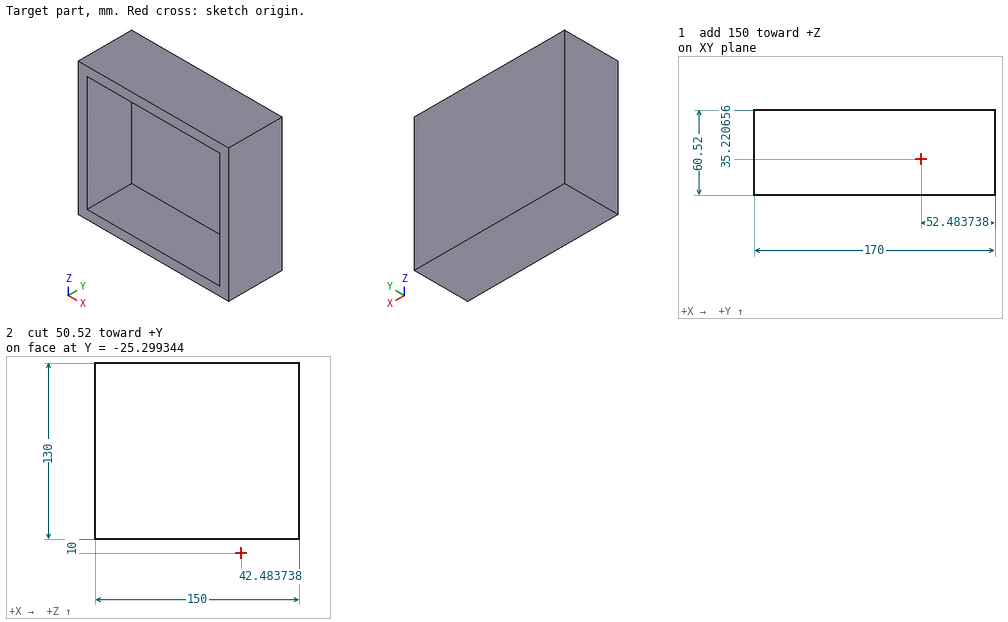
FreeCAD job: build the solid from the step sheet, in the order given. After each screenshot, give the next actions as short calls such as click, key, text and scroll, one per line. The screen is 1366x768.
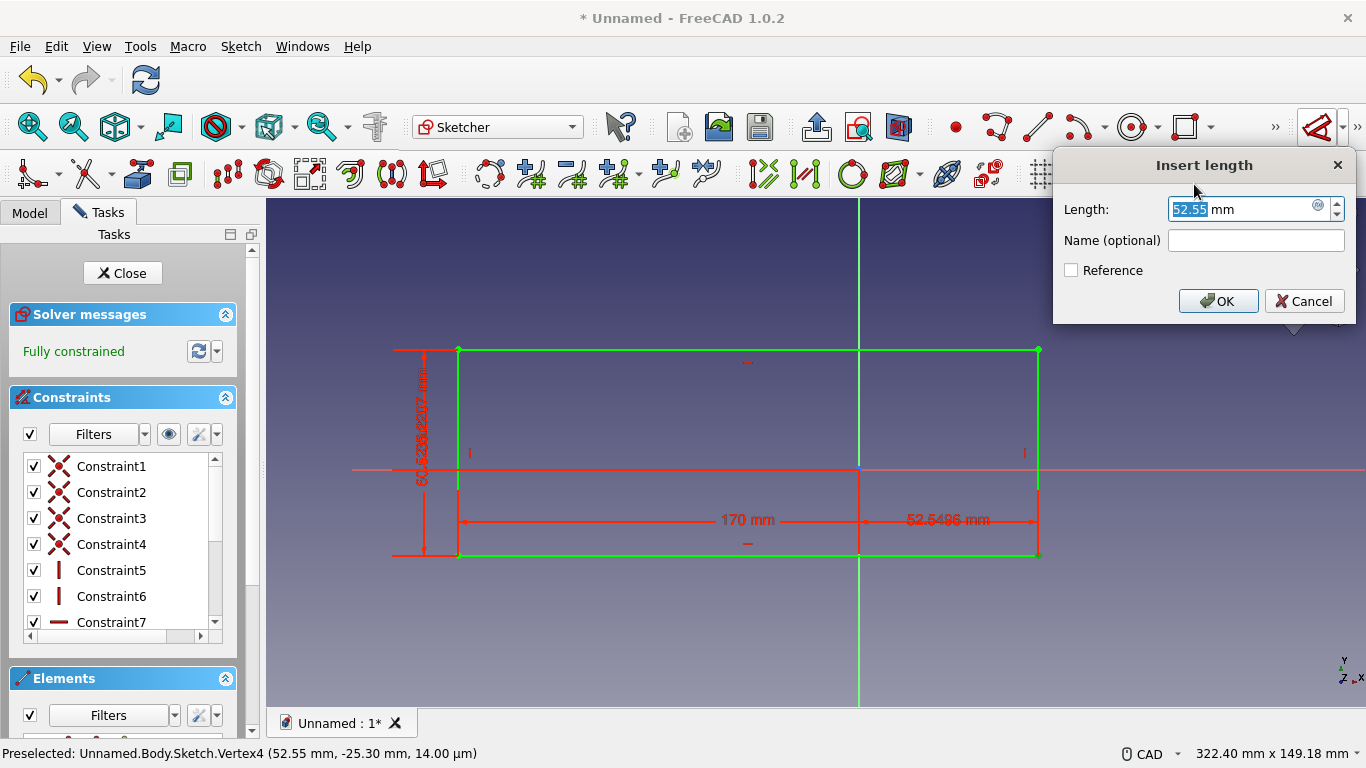
text(52.483738)
key(Return)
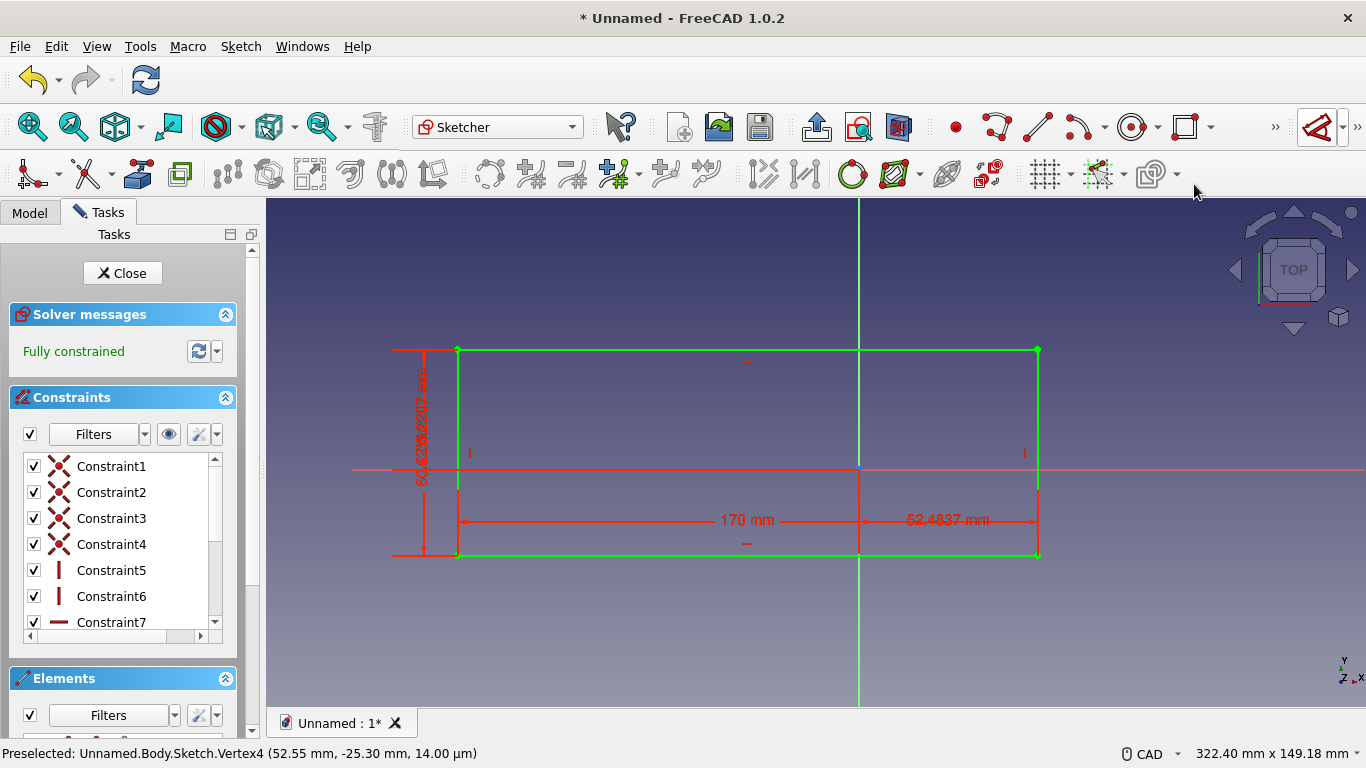
click(123, 273)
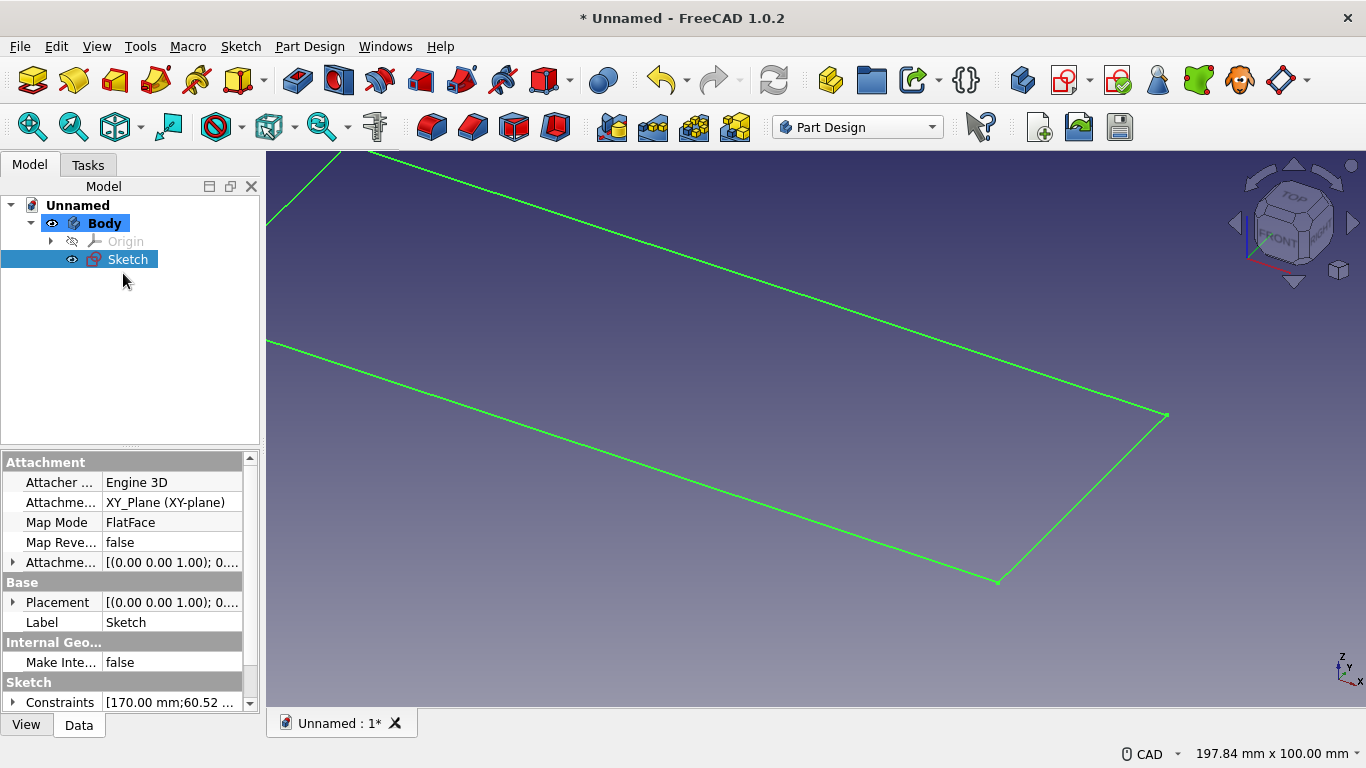
click(33, 80)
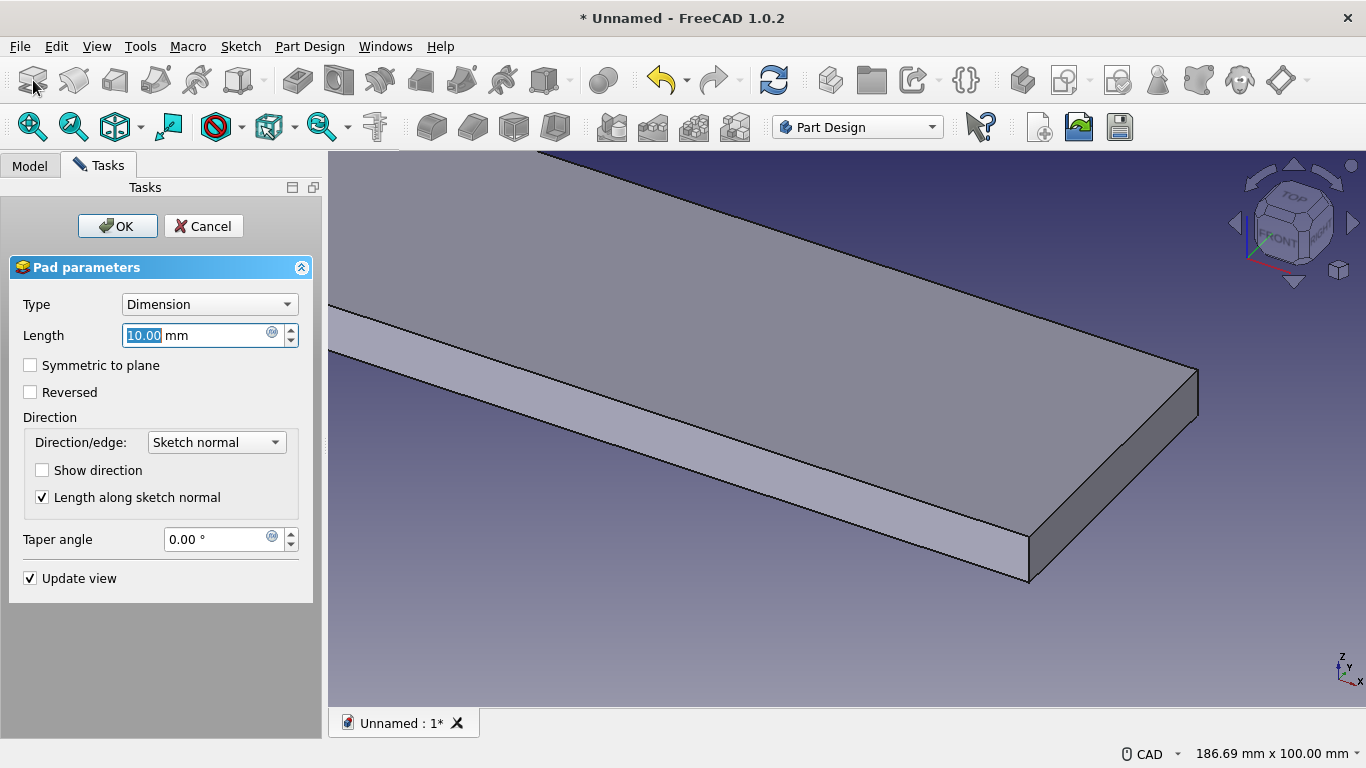
text(150)
key(Tab)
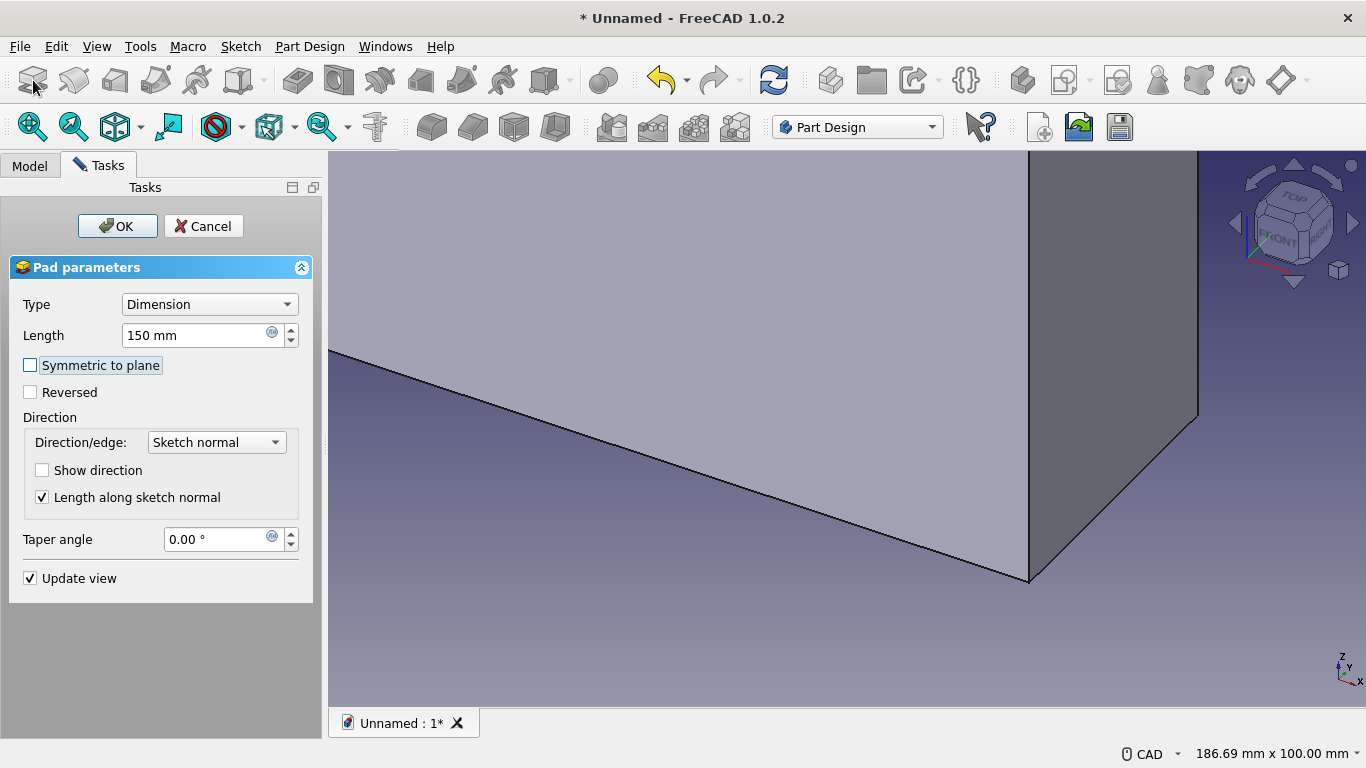
click(118, 226)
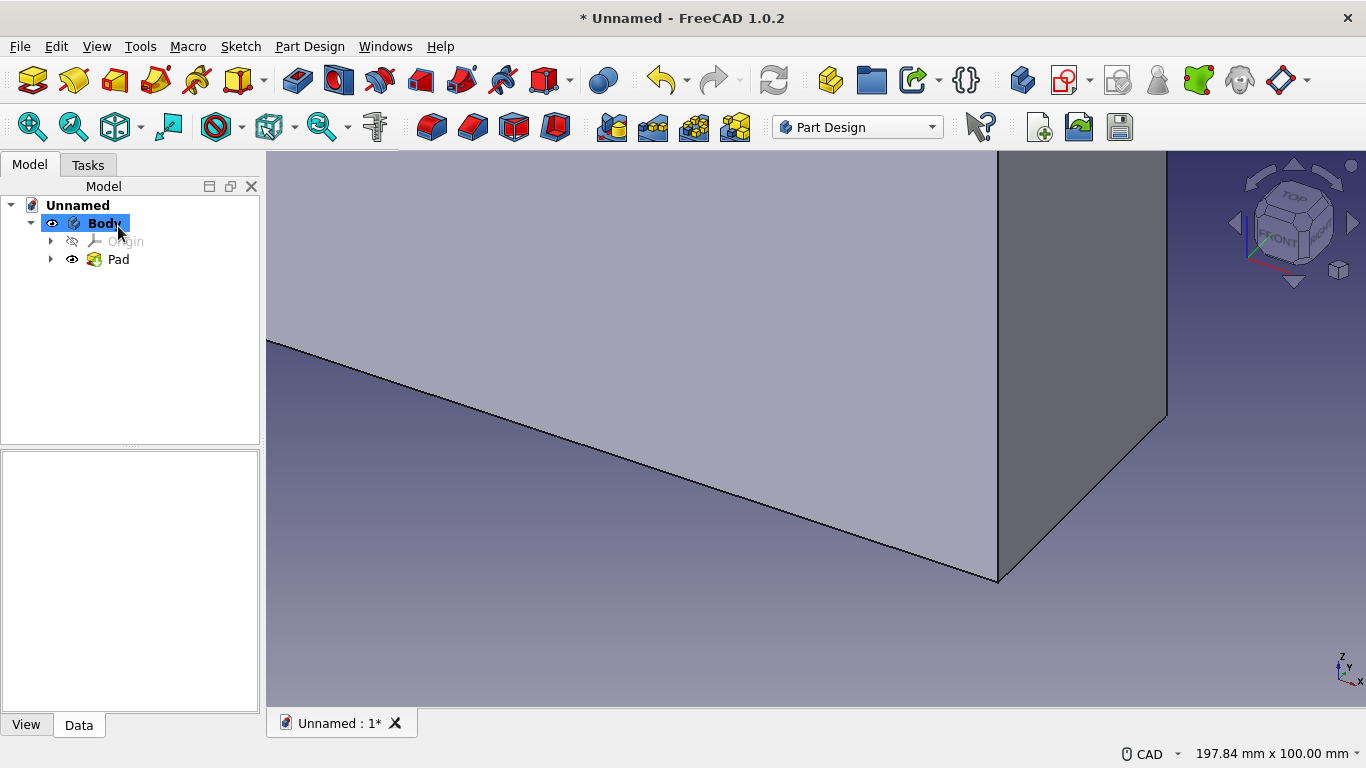
click(33, 128)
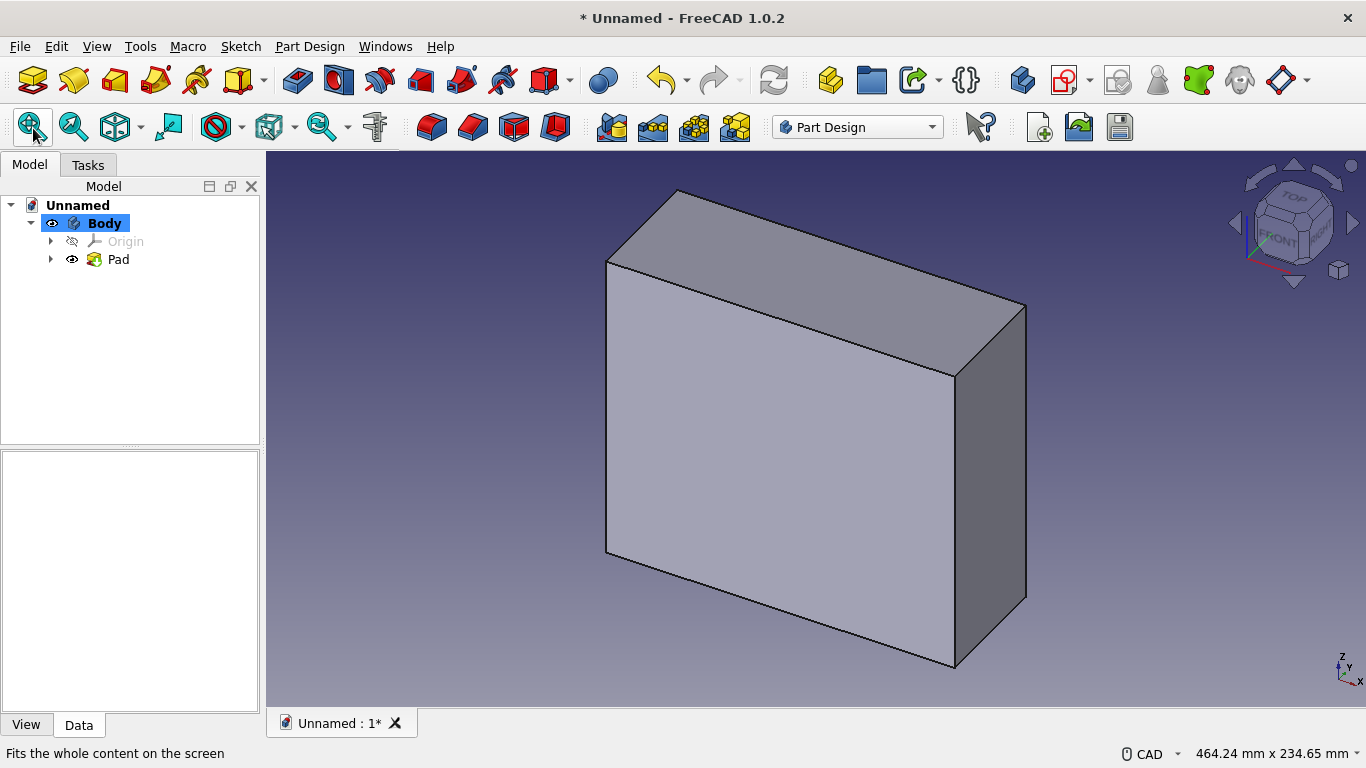
click(780, 464)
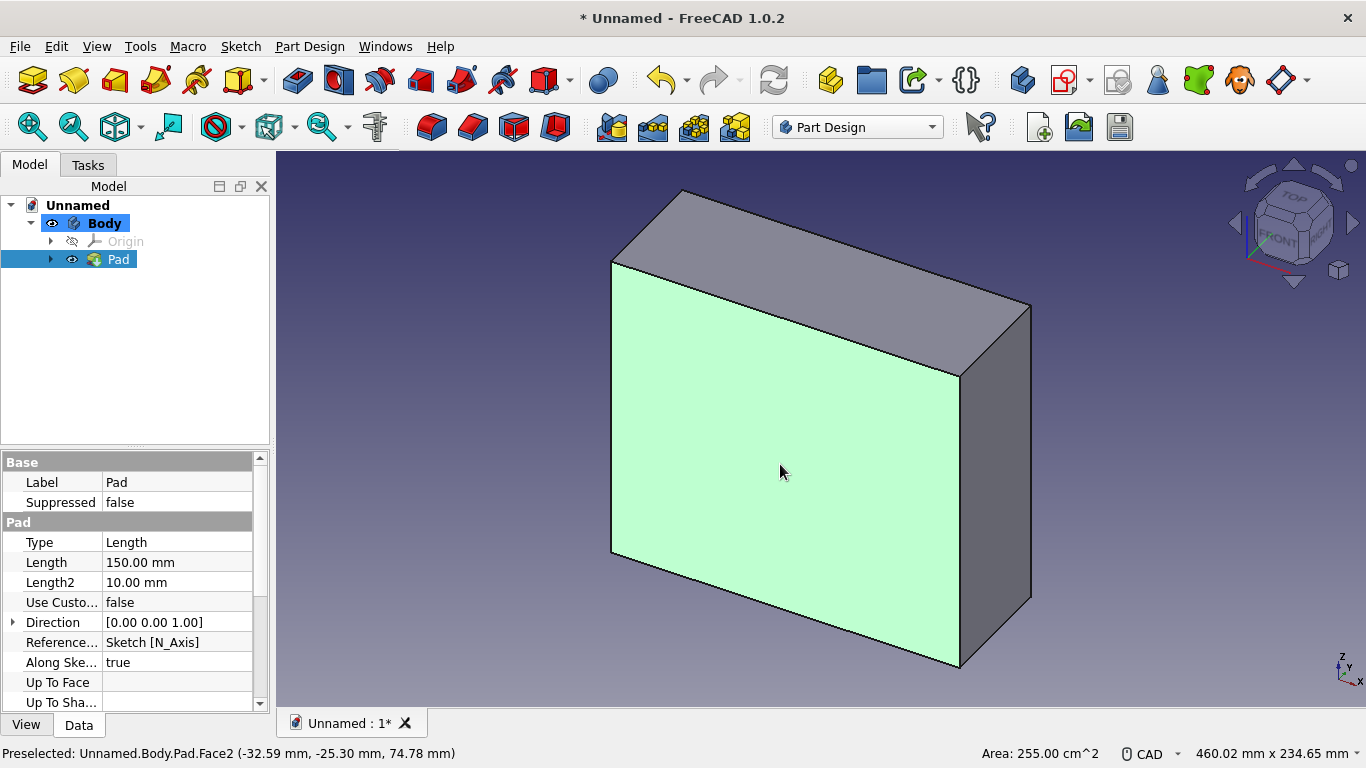
click(1064, 80)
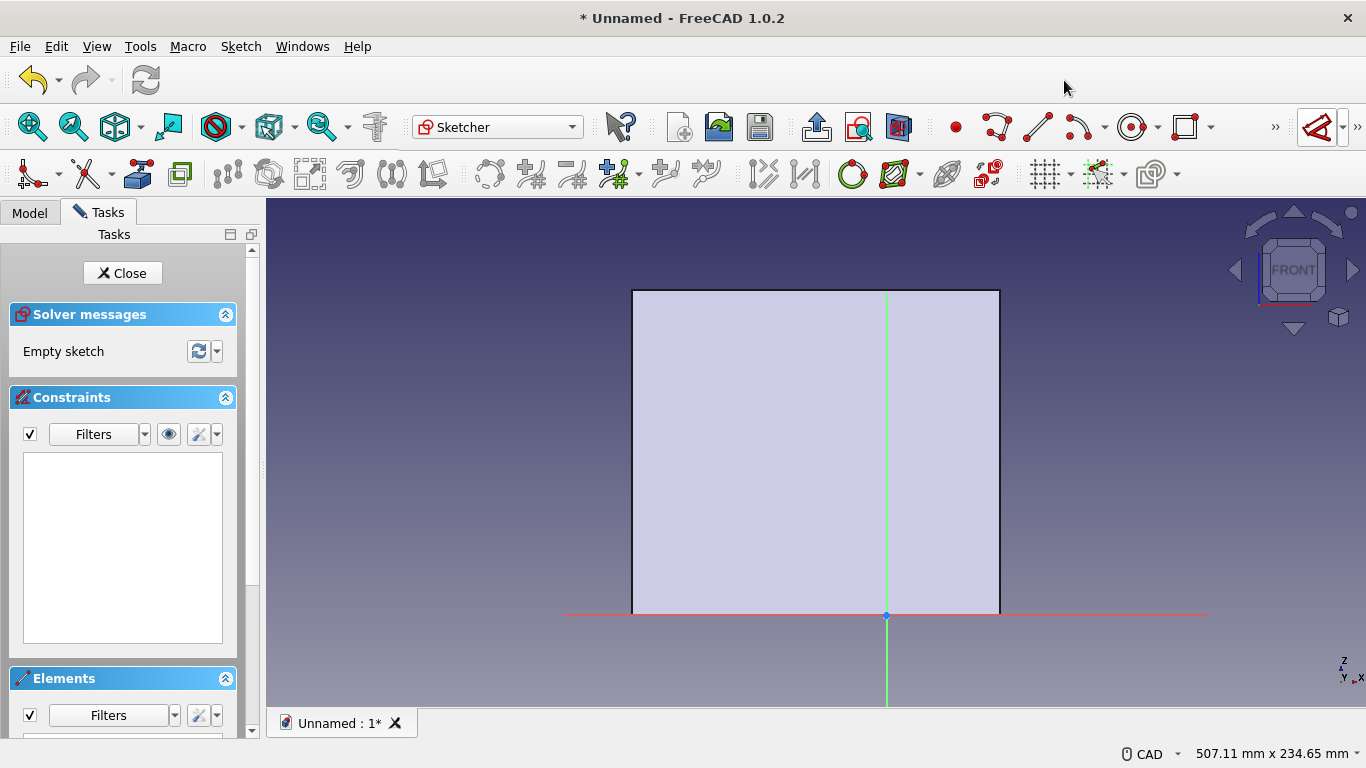
click(1184, 128)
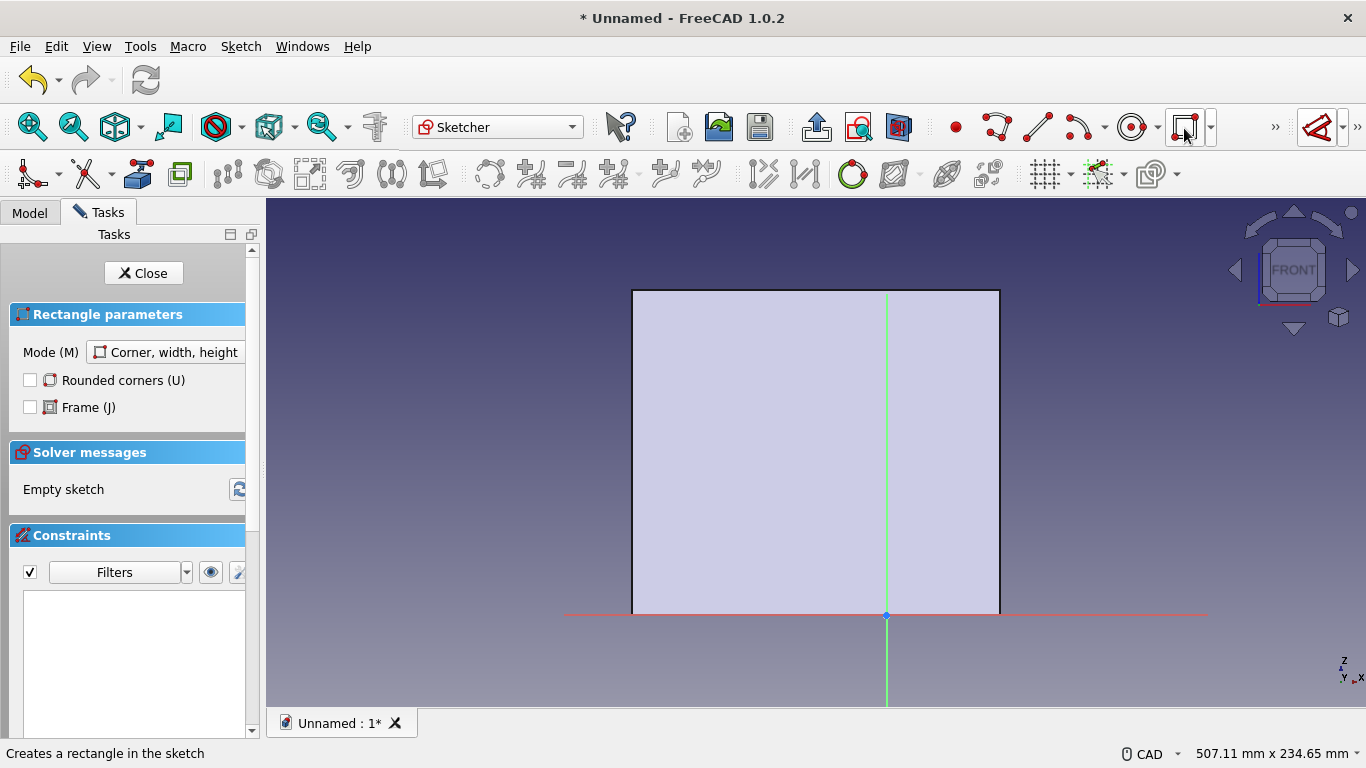
click(653, 312)
click(979, 593)
key(Escape)